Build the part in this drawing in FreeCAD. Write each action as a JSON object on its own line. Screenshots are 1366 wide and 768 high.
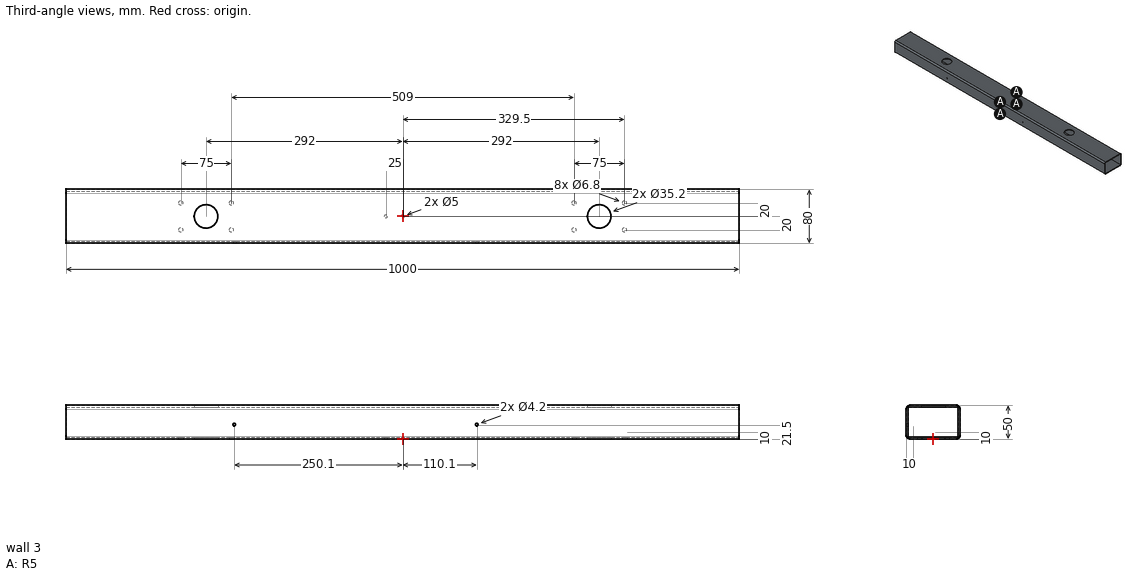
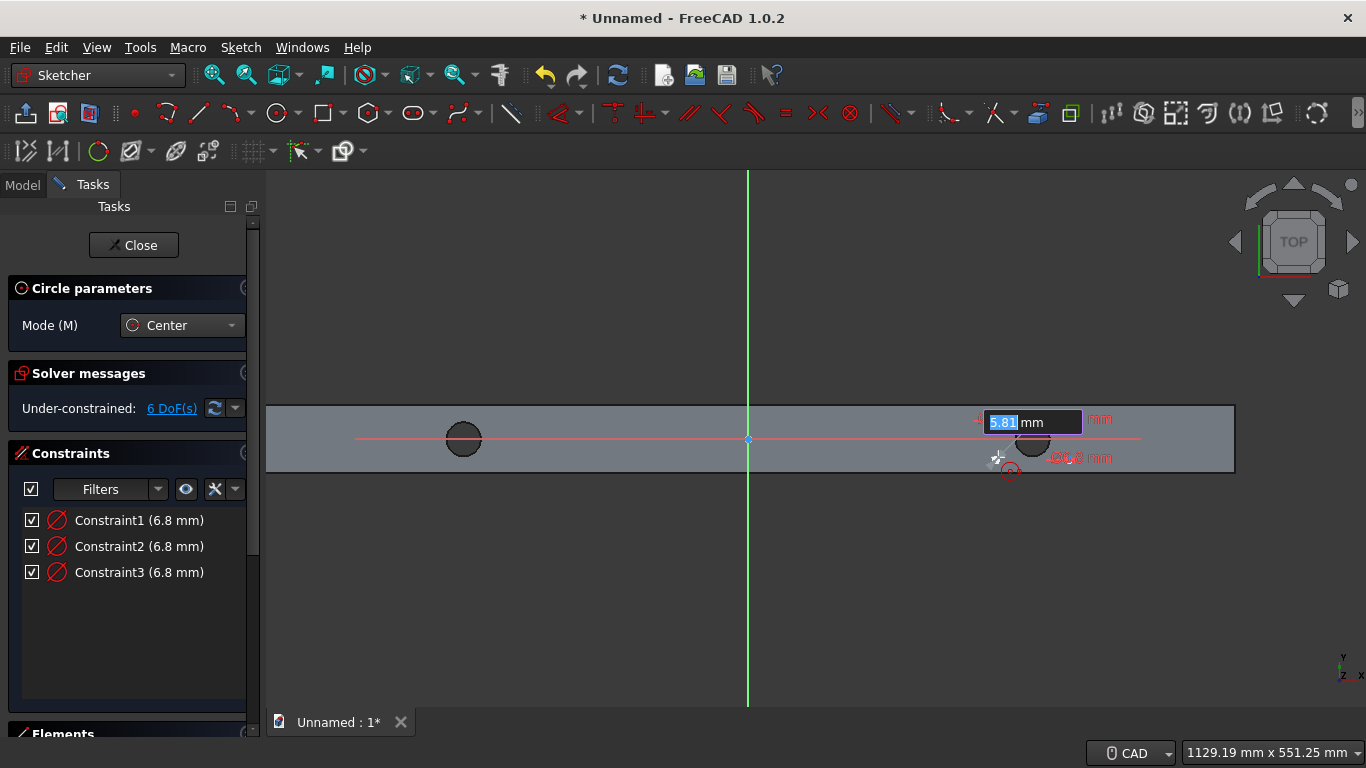
{"action": "type", "text": "6.8"}
{"action": "key", "text": "Return"}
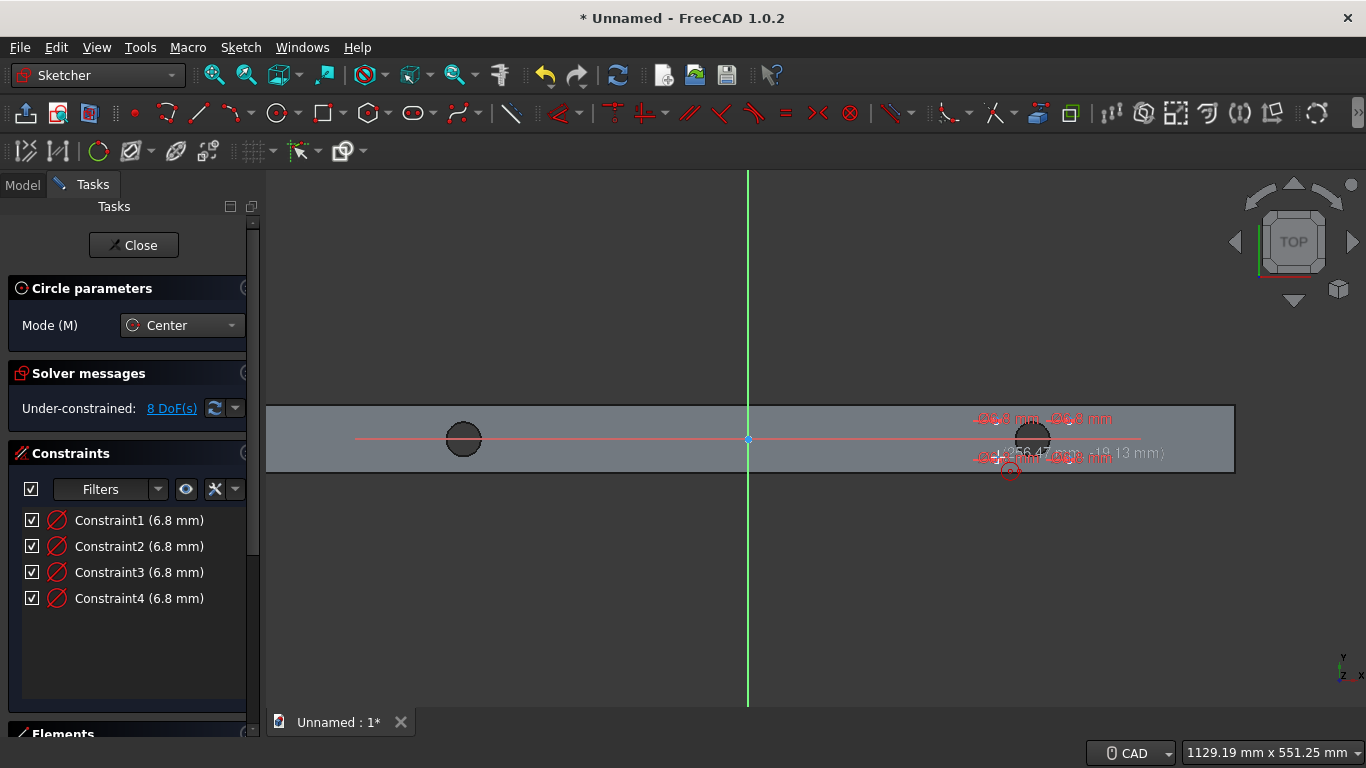
{"action": "scroll", "coordinate": [500, 420], "scroll_direction": "up", "scroll_amount": 10}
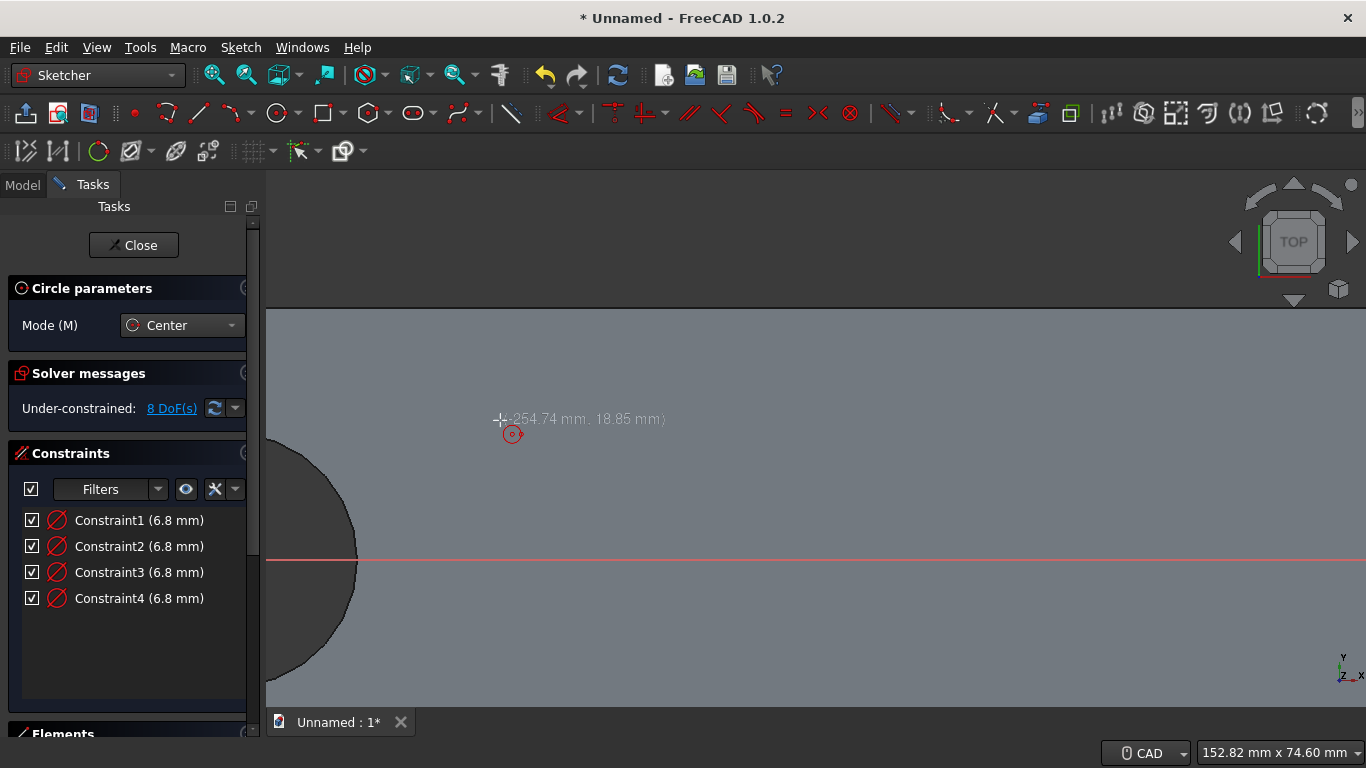
{"action": "scroll", "coordinate": [499, 419], "scroll_direction": "down", "scroll_amount": 10}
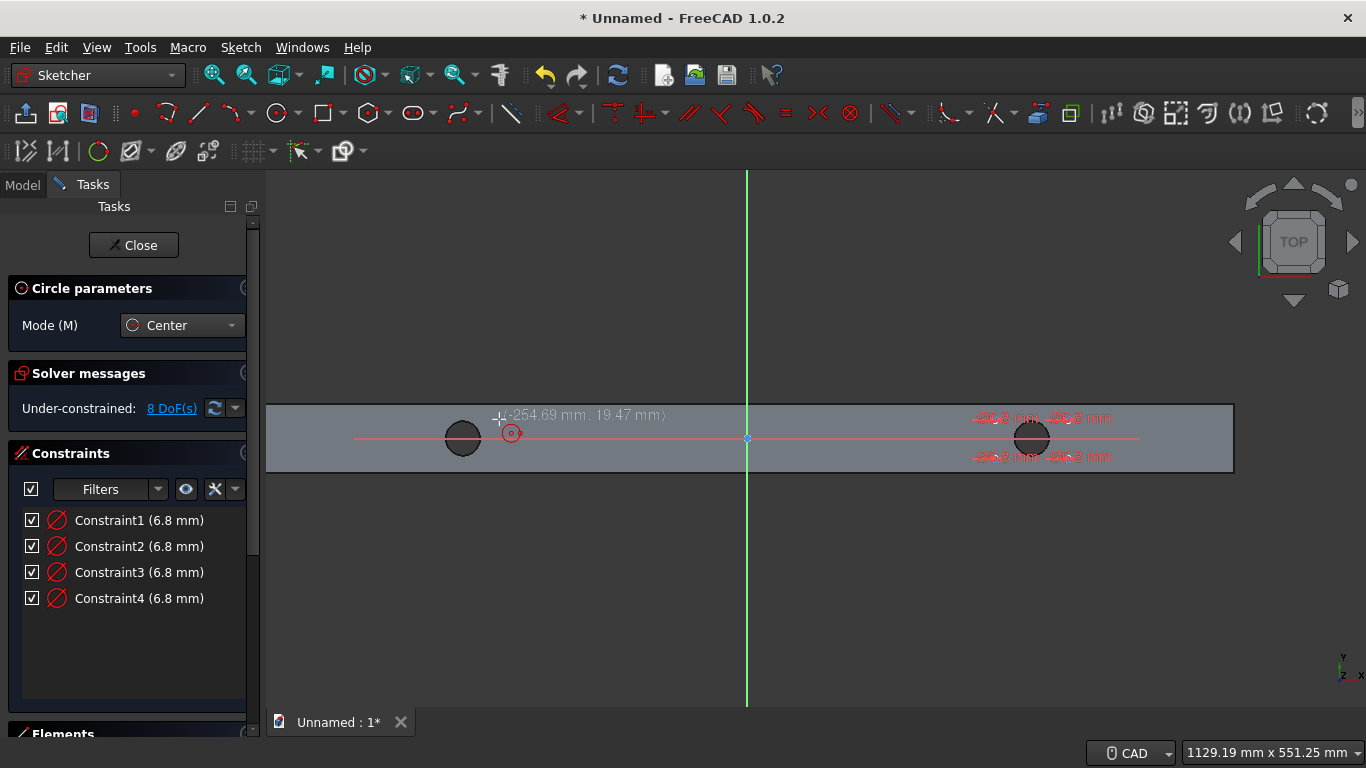
{"action": "left_click", "coordinate": [499, 419]}
{"action": "mouse_move", "coordinate": [502, 417]}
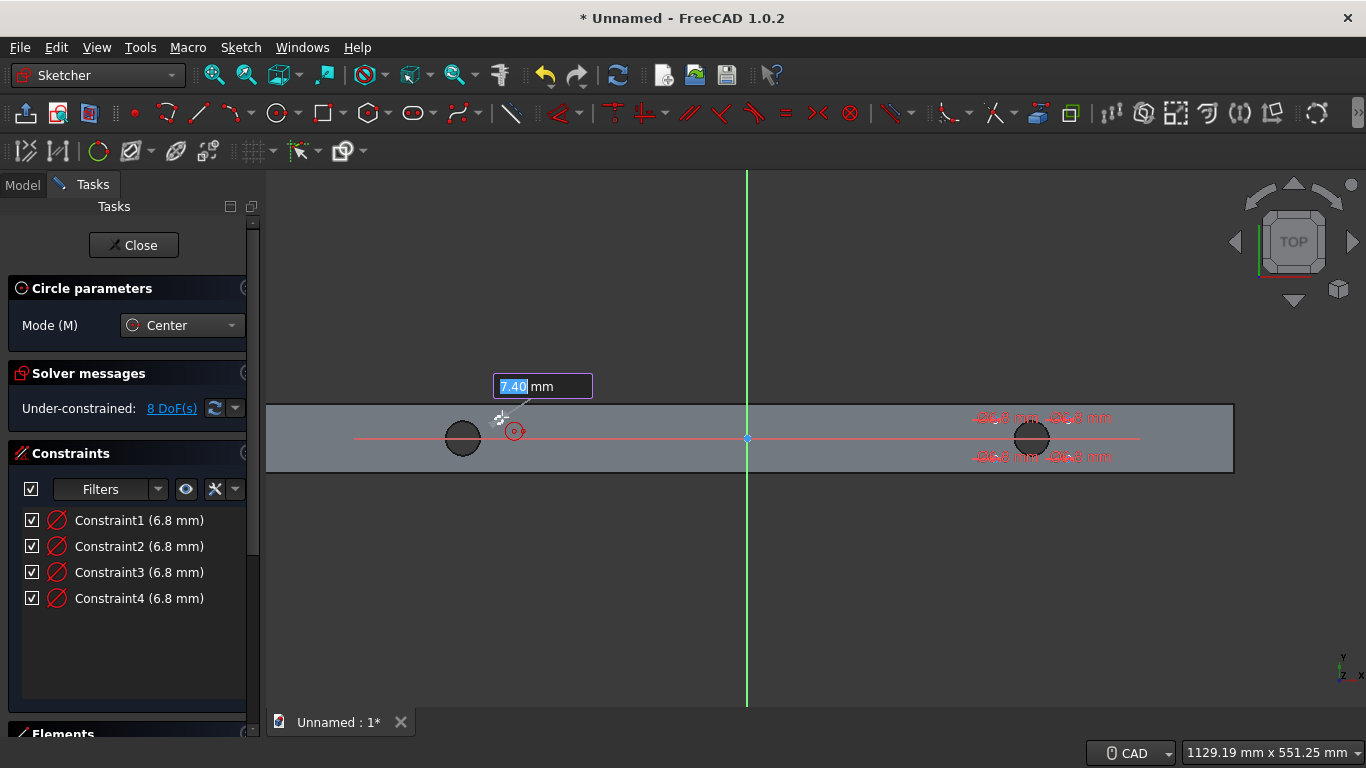
{"action": "type", "text": "6.8"}
{"action": "key", "text": "Return"}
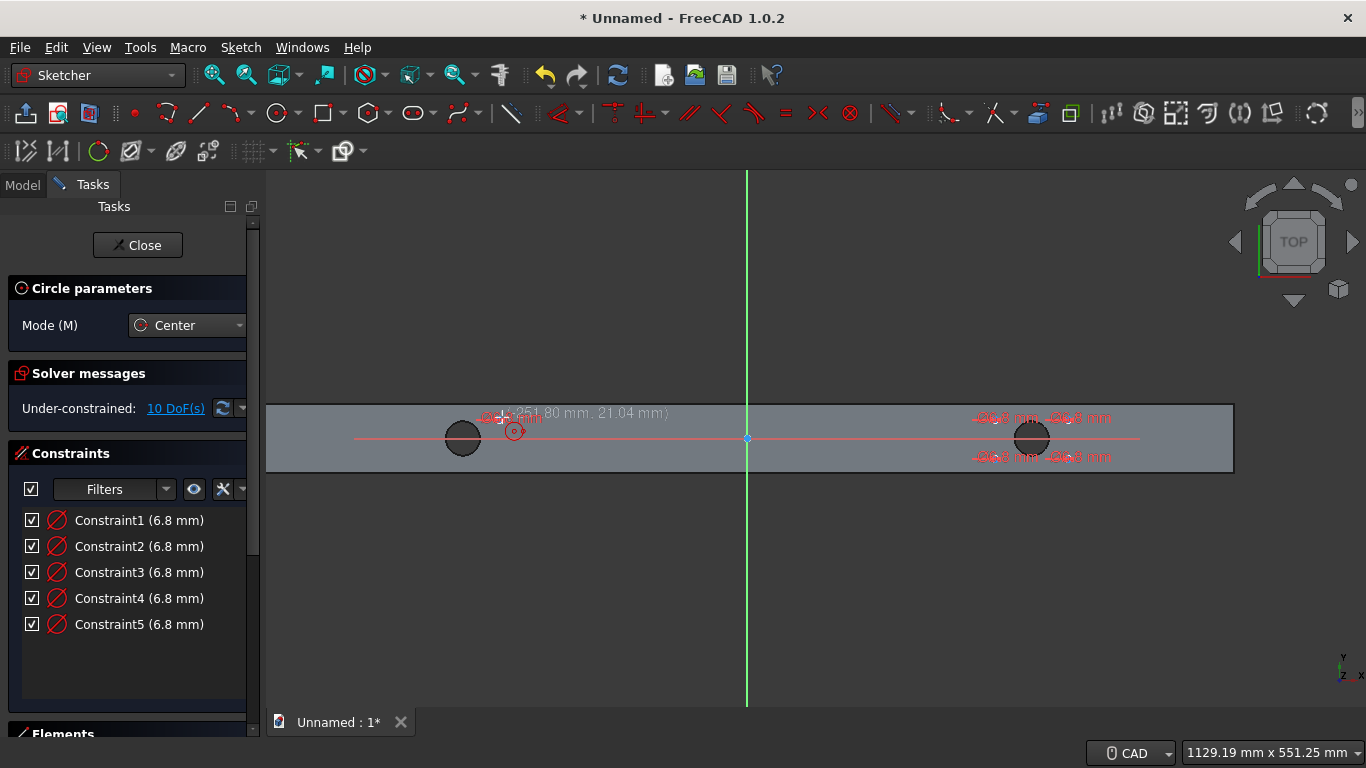
{"action": "scroll", "coordinate": [499, 458], "scroll_direction": "up", "scroll_amount": 10}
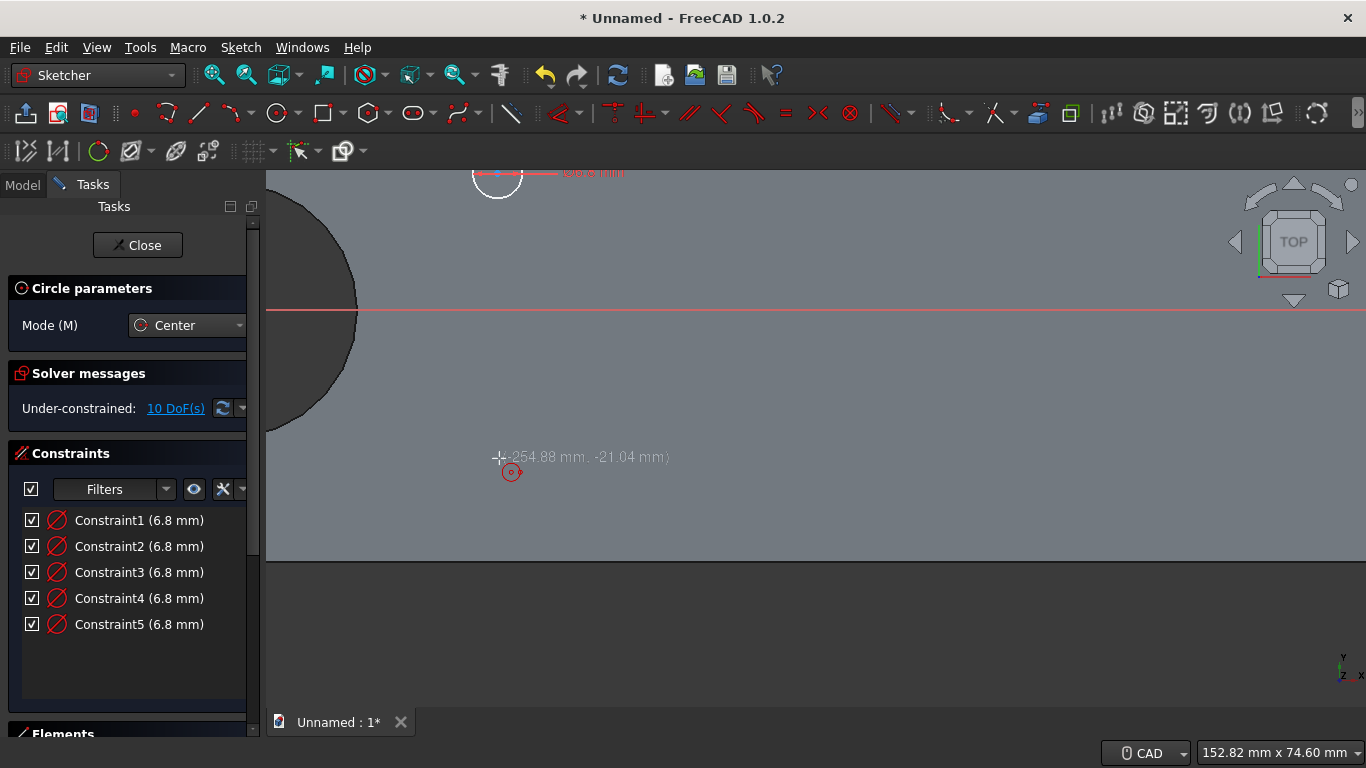
{"action": "scroll", "coordinate": [499, 459], "scroll_direction": "down", "scroll_amount": 10}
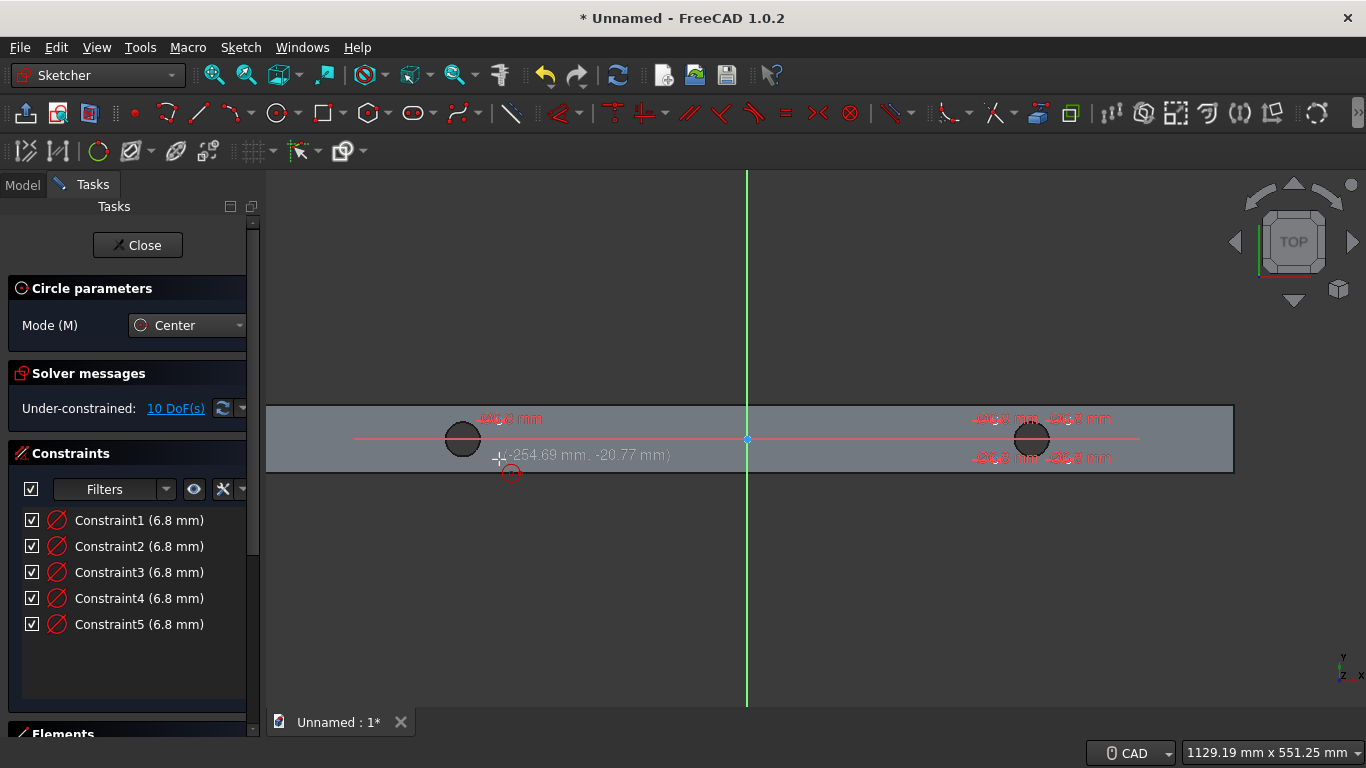
{"action": "left_click", "coordinate": [499, 459]}
{"action": "mouse_move", "coordinate": [502, 457]}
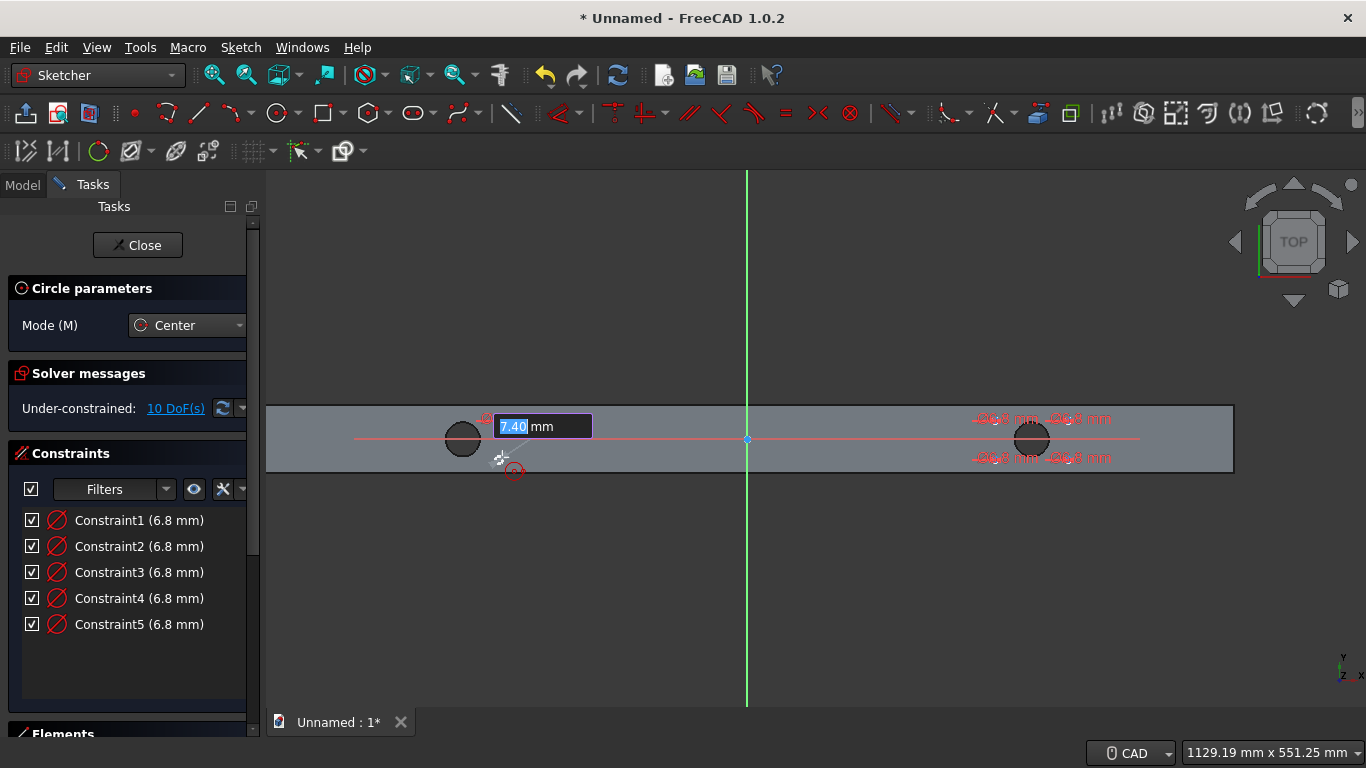
{"action": "type", "text": "6.8"}
{"action": "key", "text": "Return"}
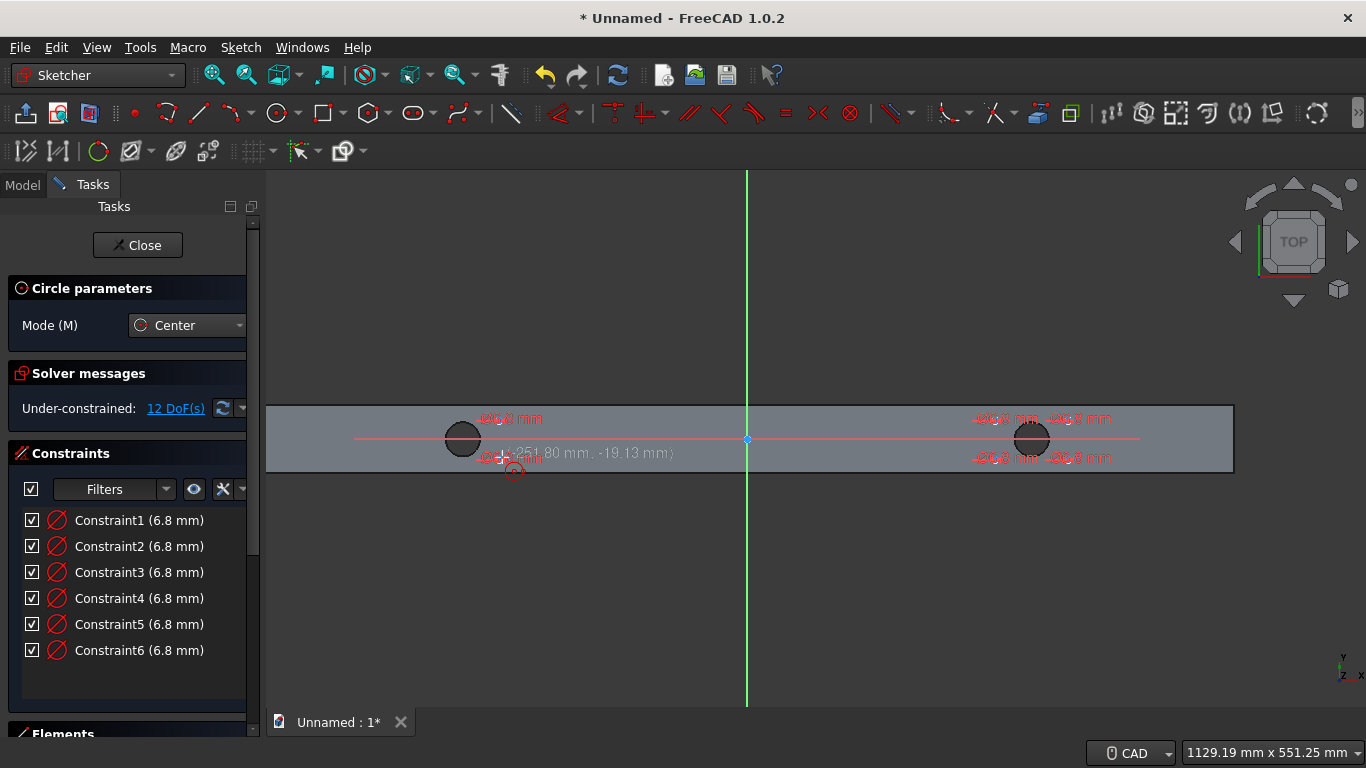
{"action": "scroll", "coordinate": [426, 420], "scroll_direction": "up", "scroll_amount": 10}